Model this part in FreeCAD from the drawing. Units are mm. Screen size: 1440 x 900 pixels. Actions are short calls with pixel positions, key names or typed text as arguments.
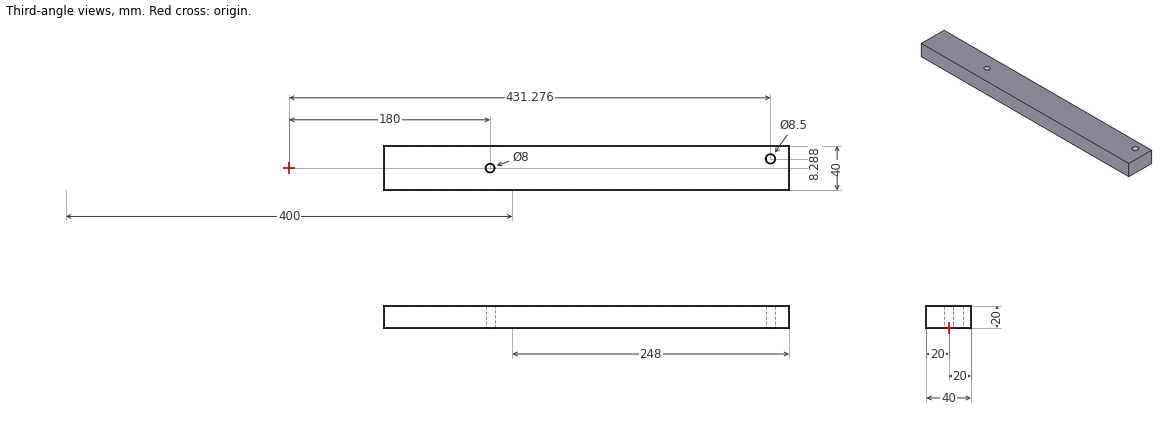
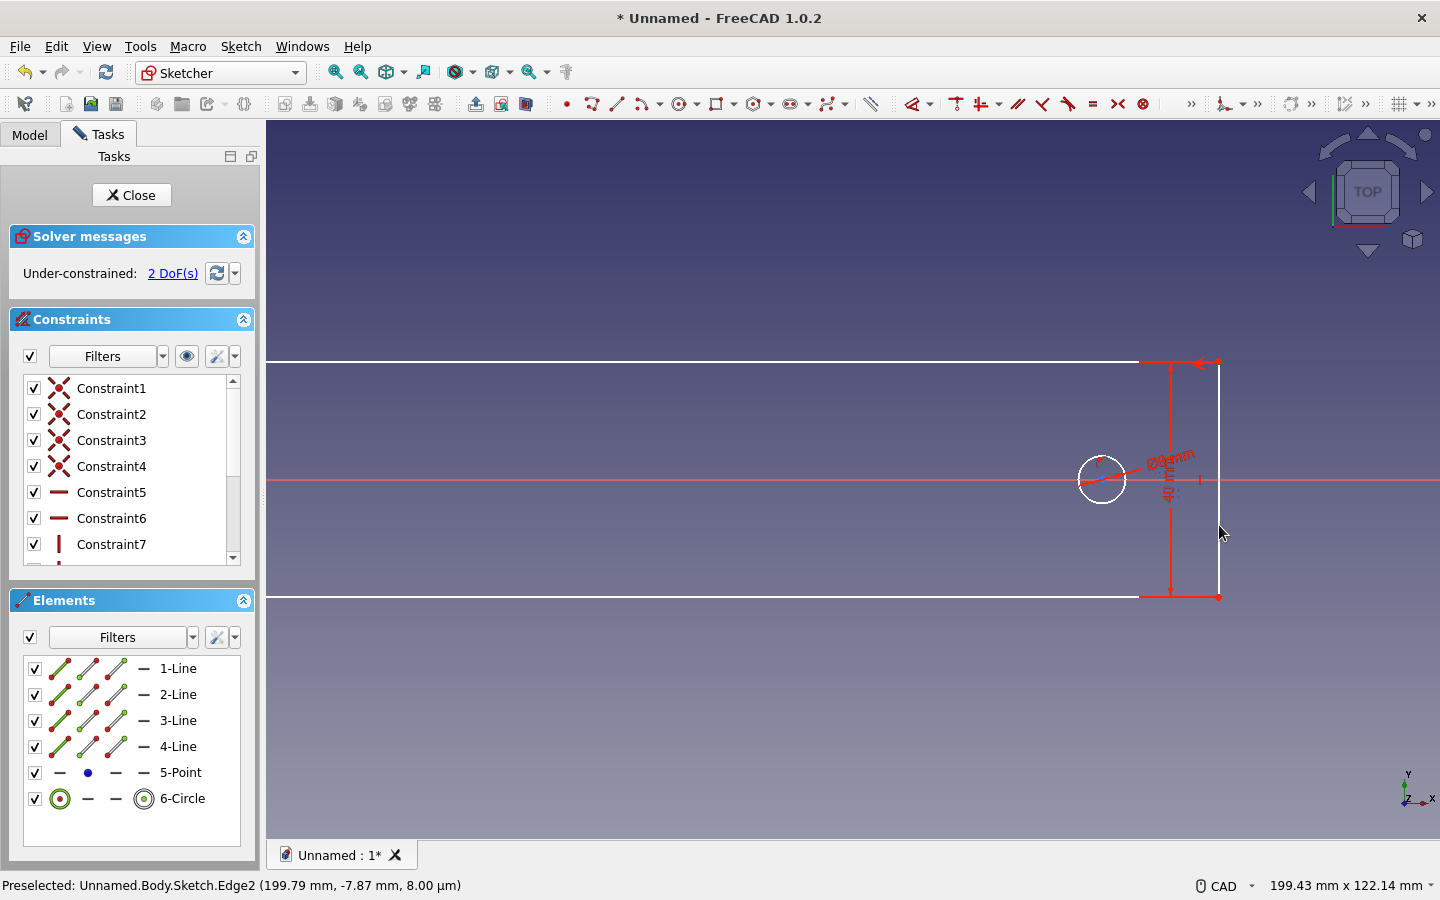
click(513, 597)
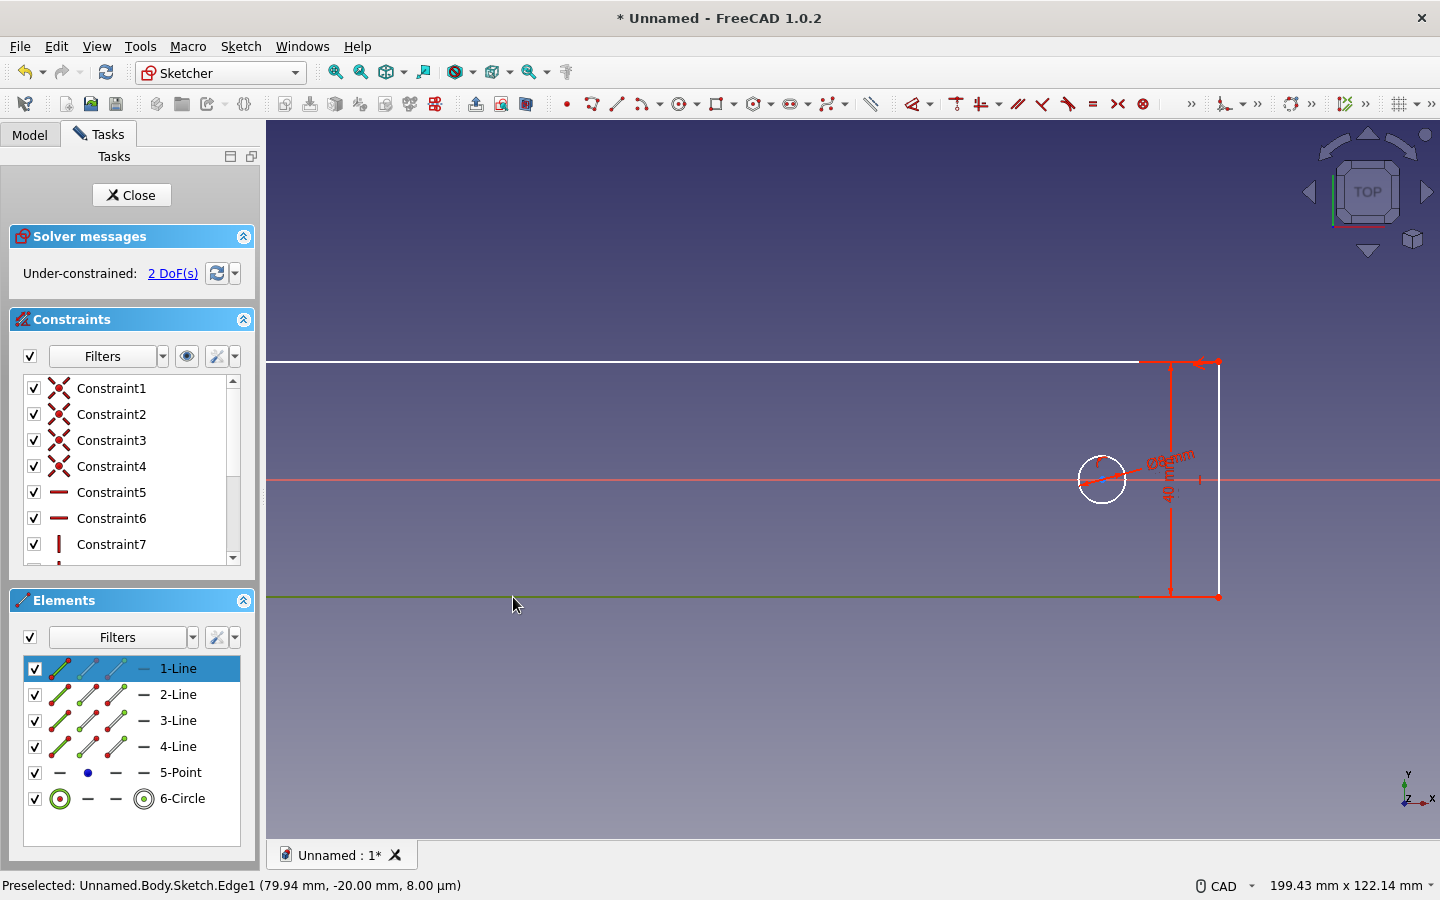
click(930, 104)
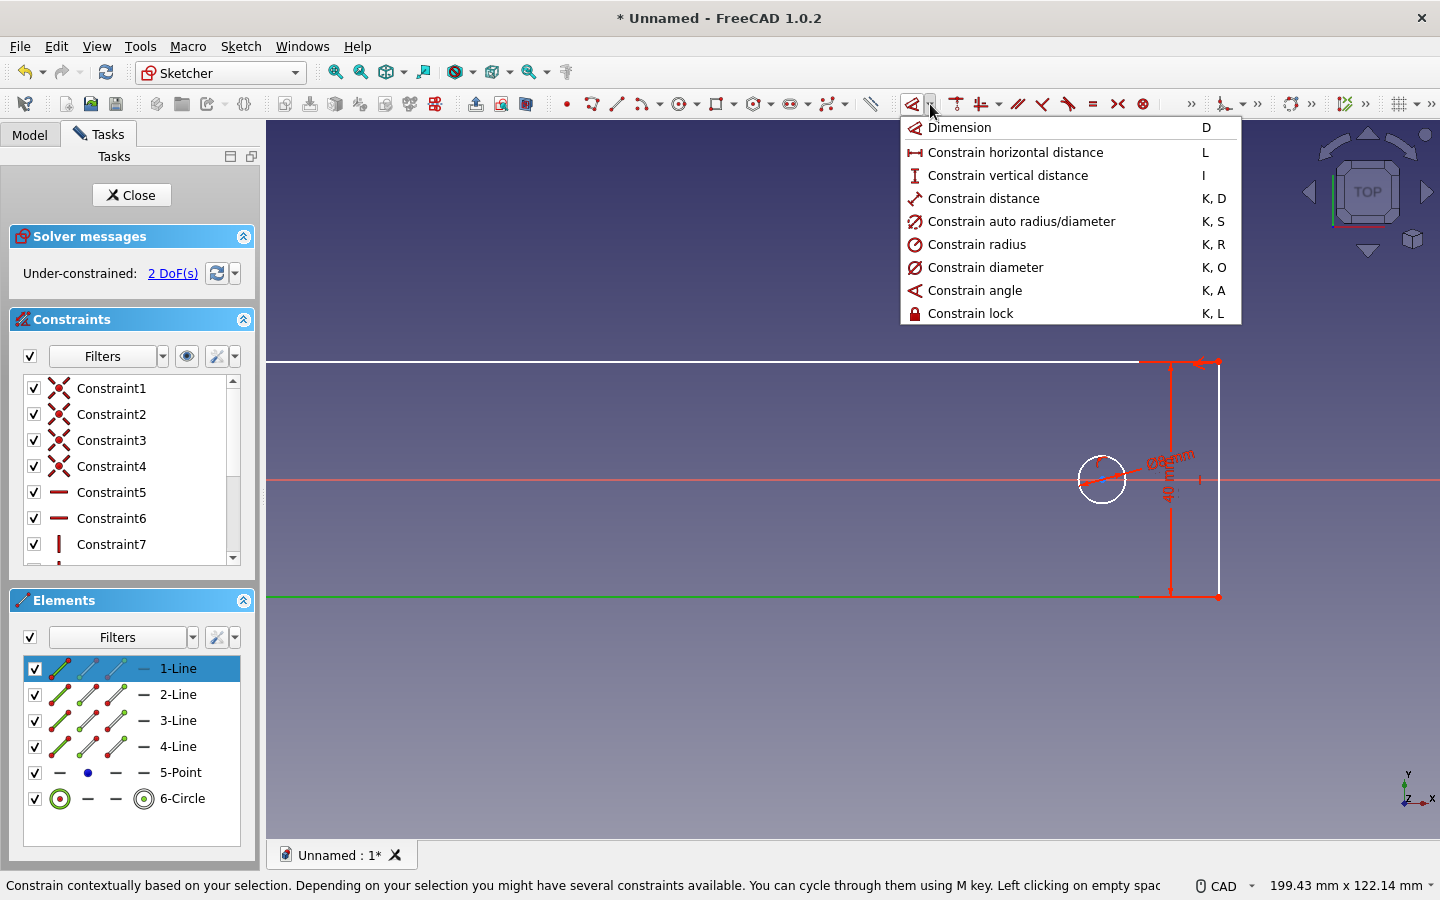
click(1071, 152)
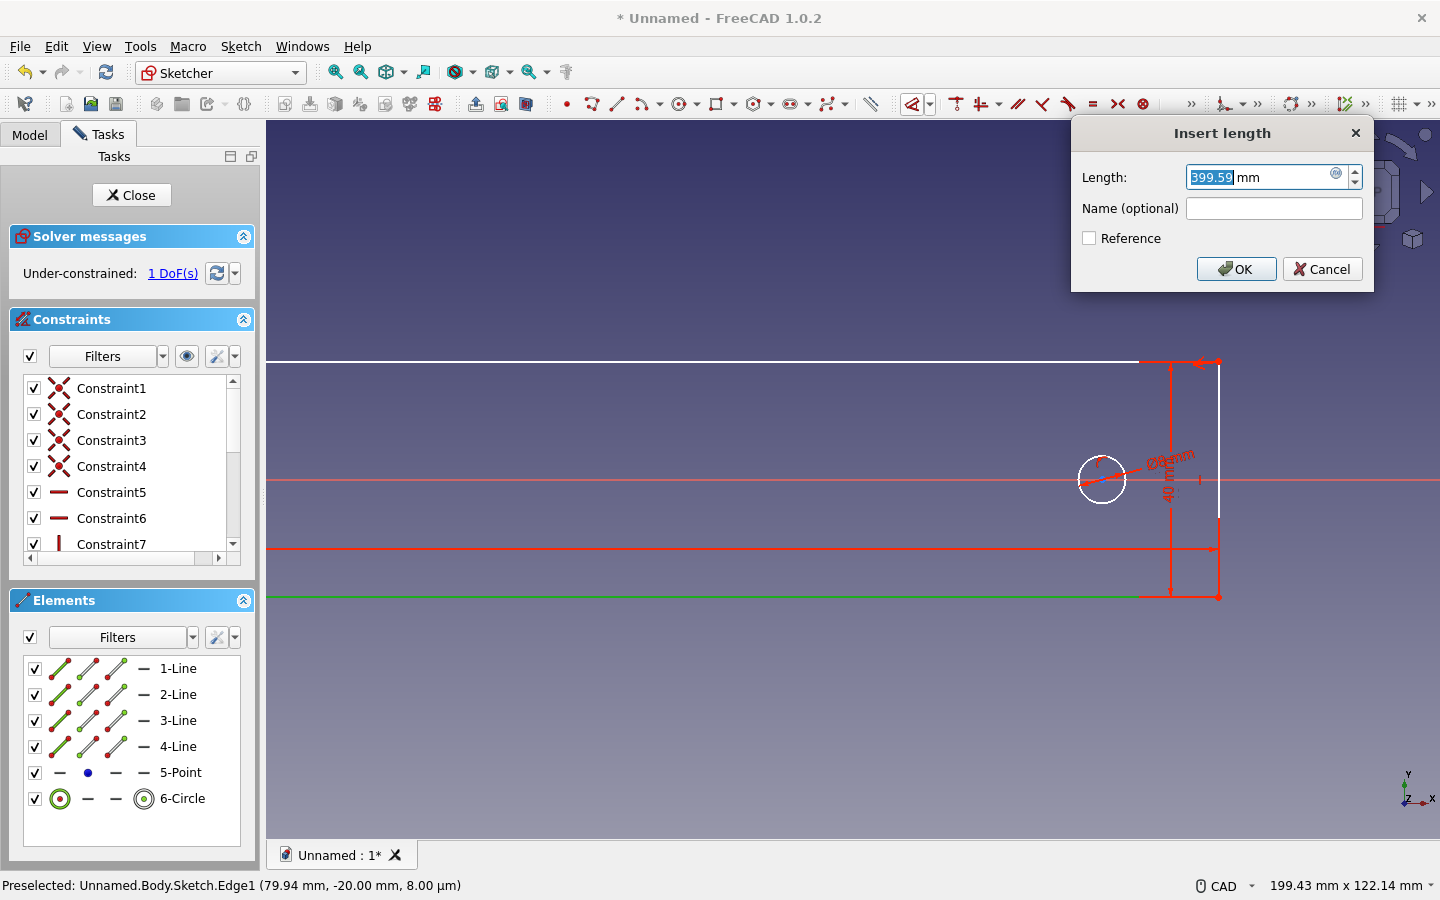
text(400)
key(Return)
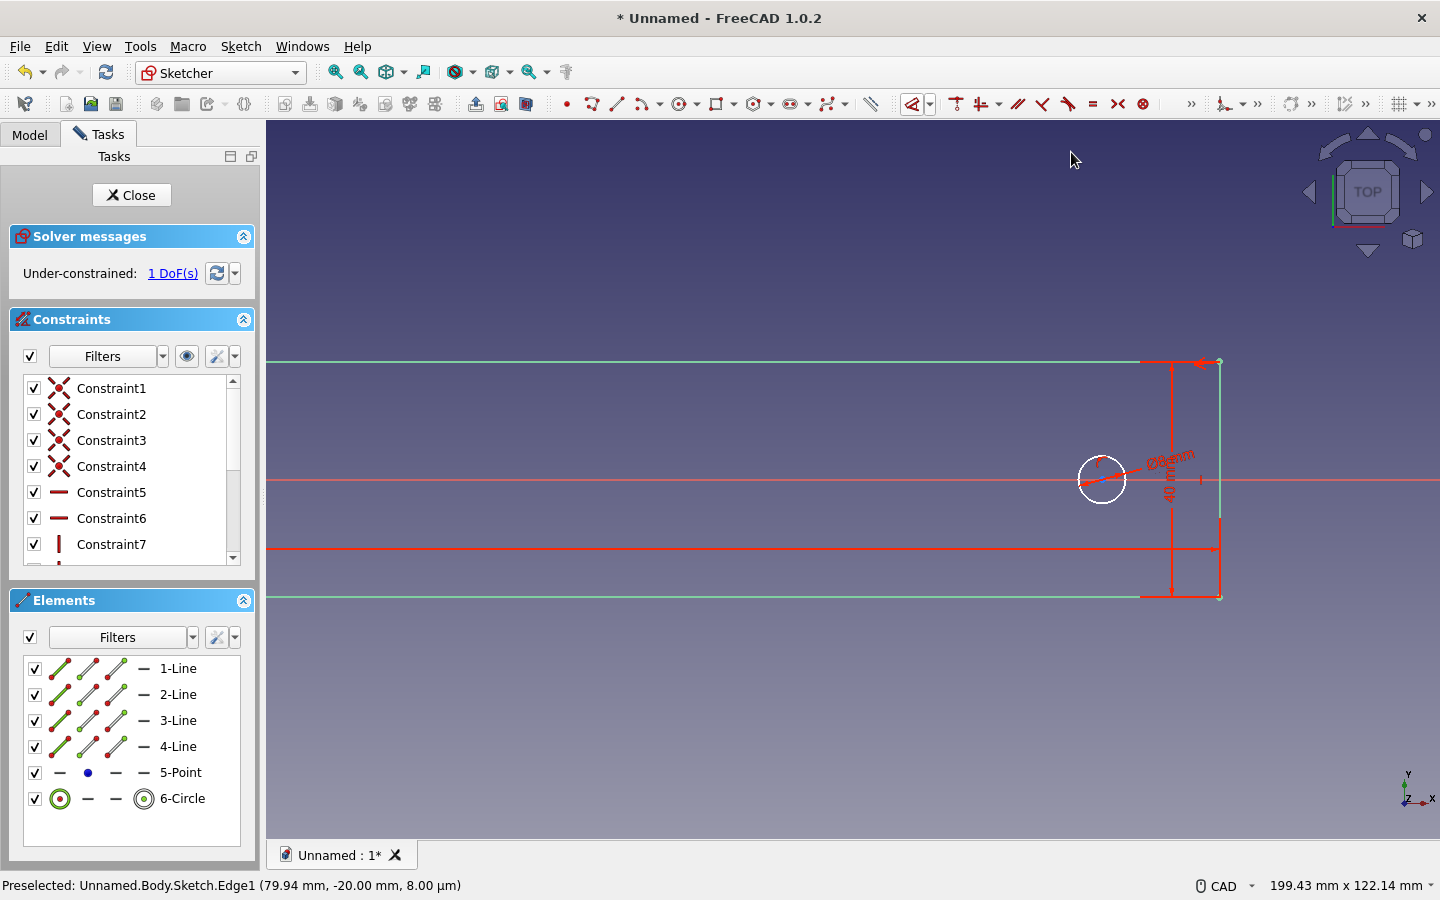
click(1102, 480)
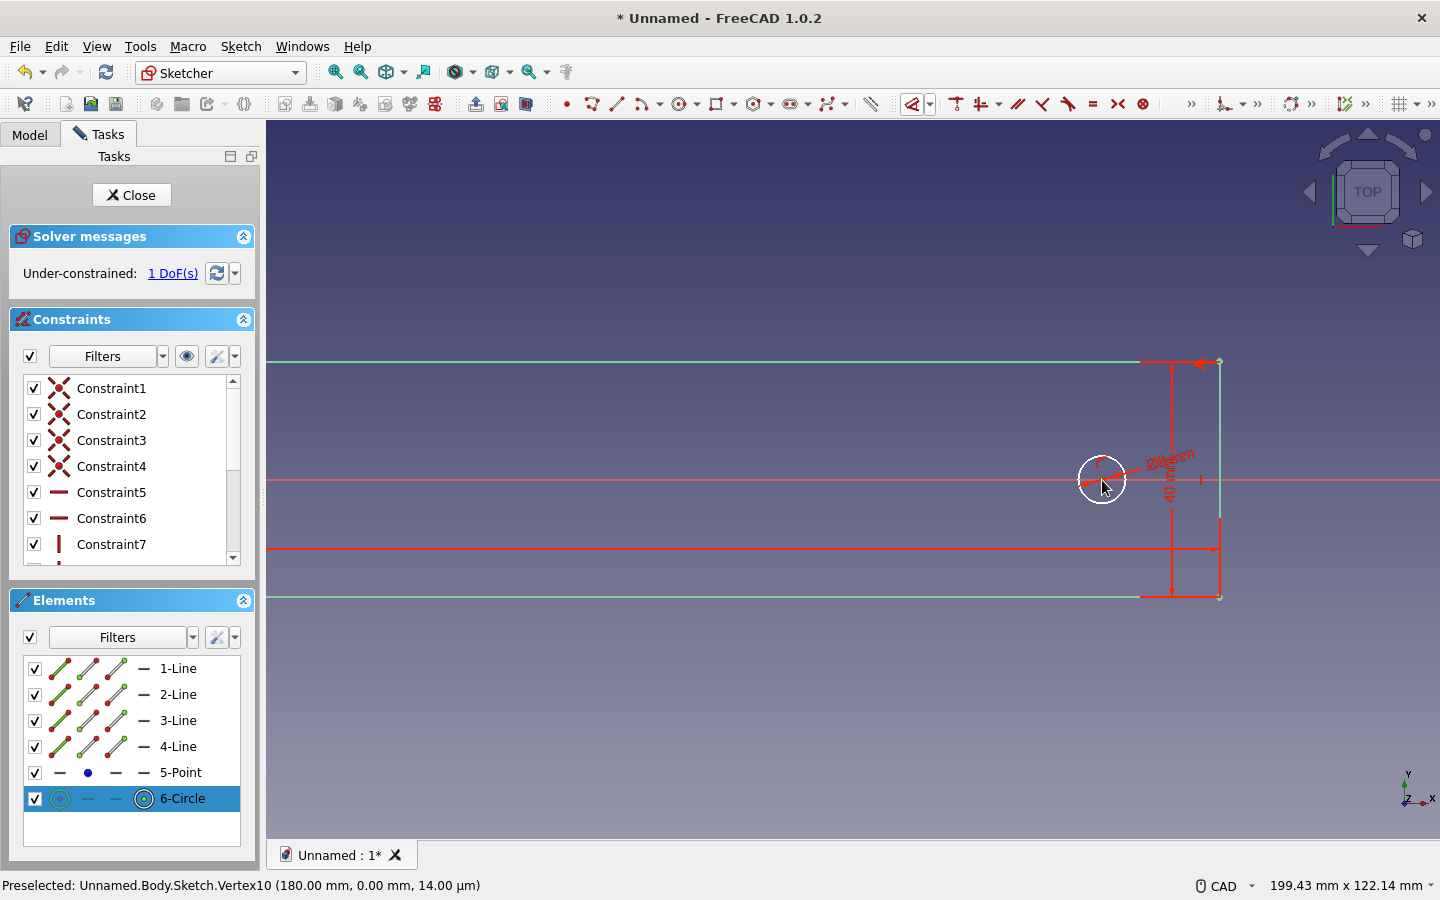
click(930, 104)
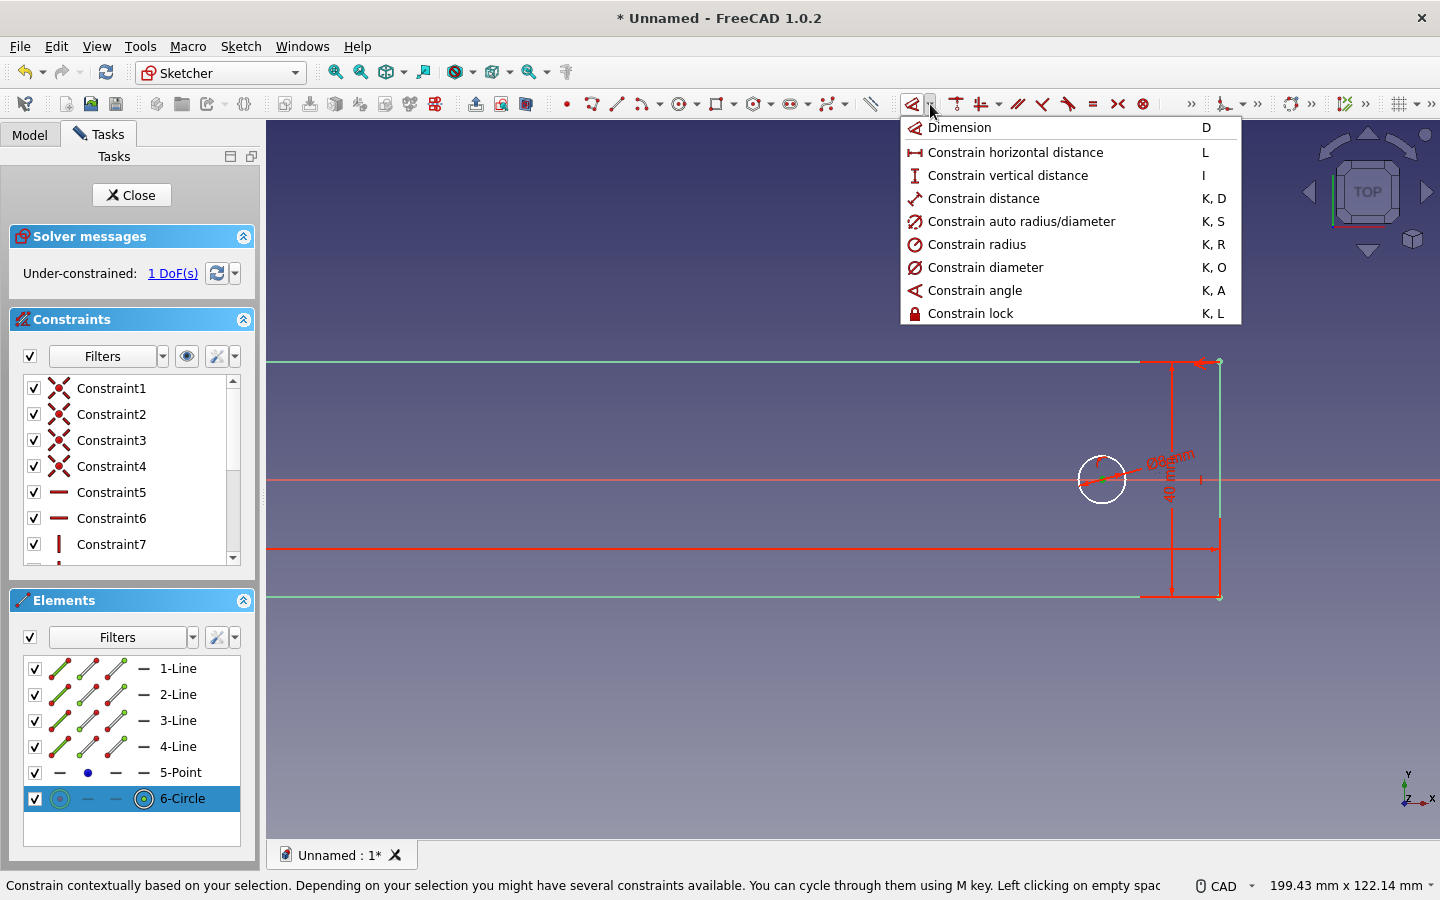
click(1071, 152)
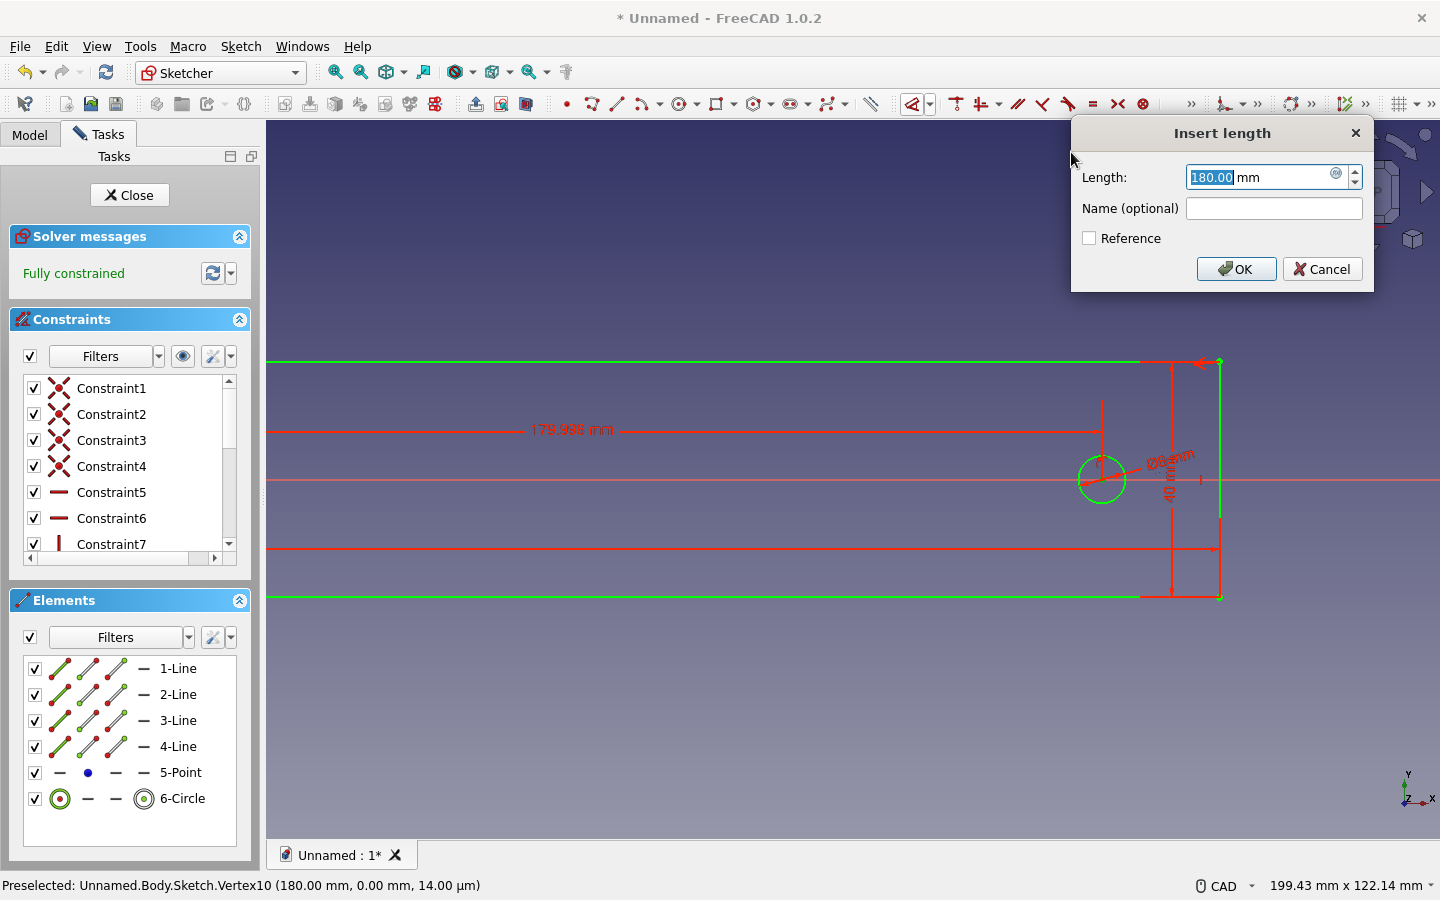
text(180)
key(Return)